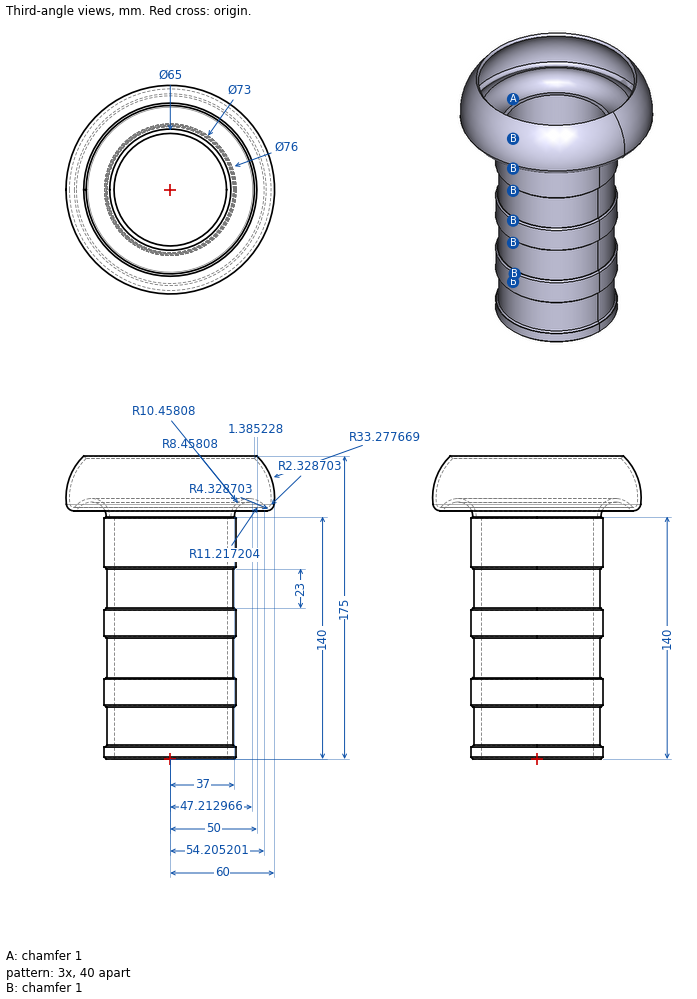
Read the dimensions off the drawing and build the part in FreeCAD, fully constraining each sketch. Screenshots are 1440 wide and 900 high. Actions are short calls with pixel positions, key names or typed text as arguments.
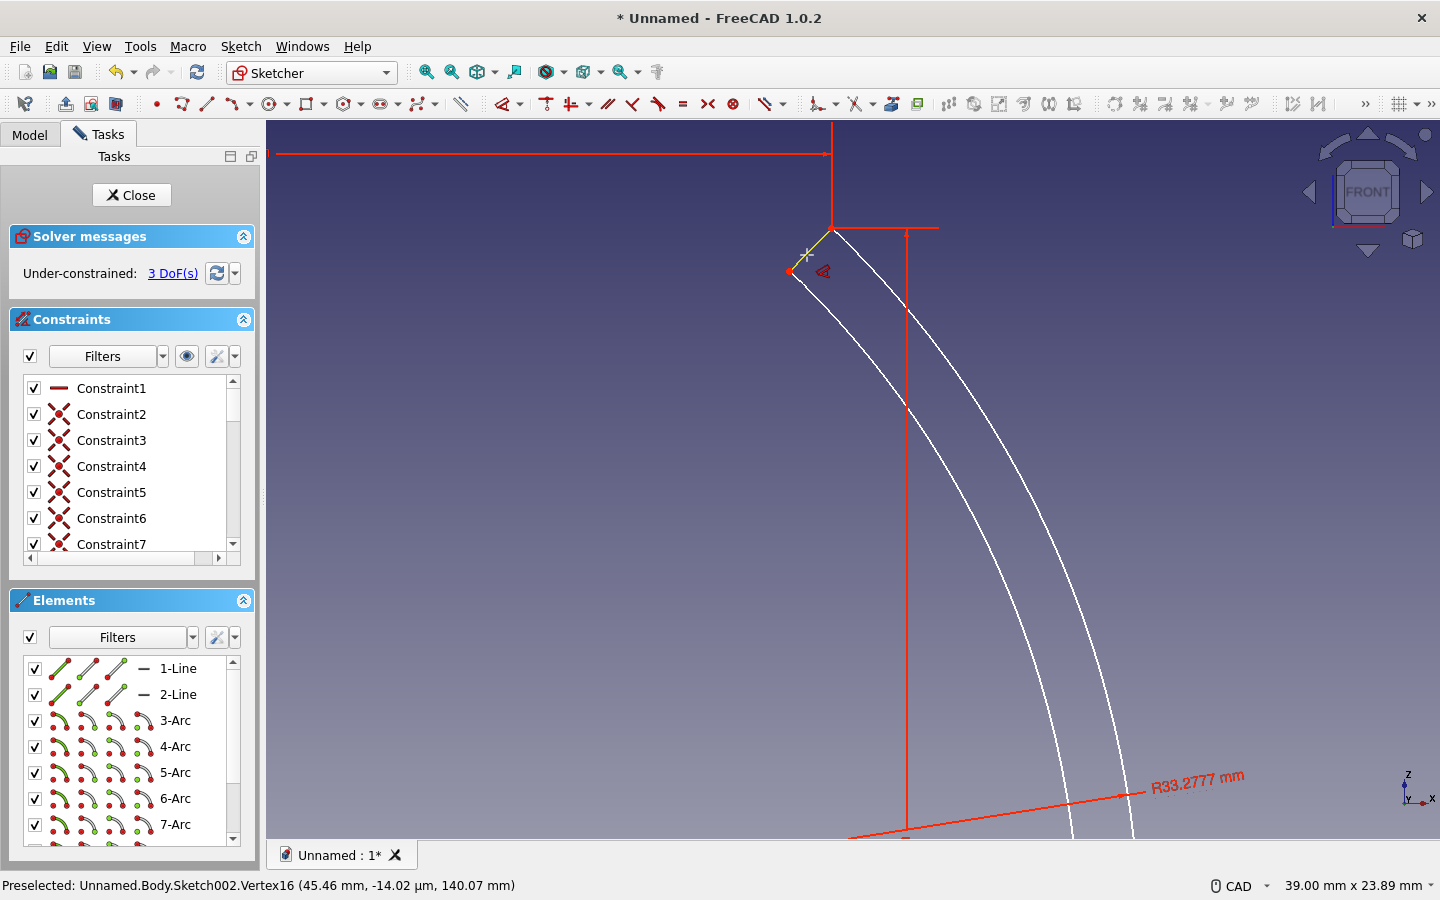
click(807, 254)
click(811, 194)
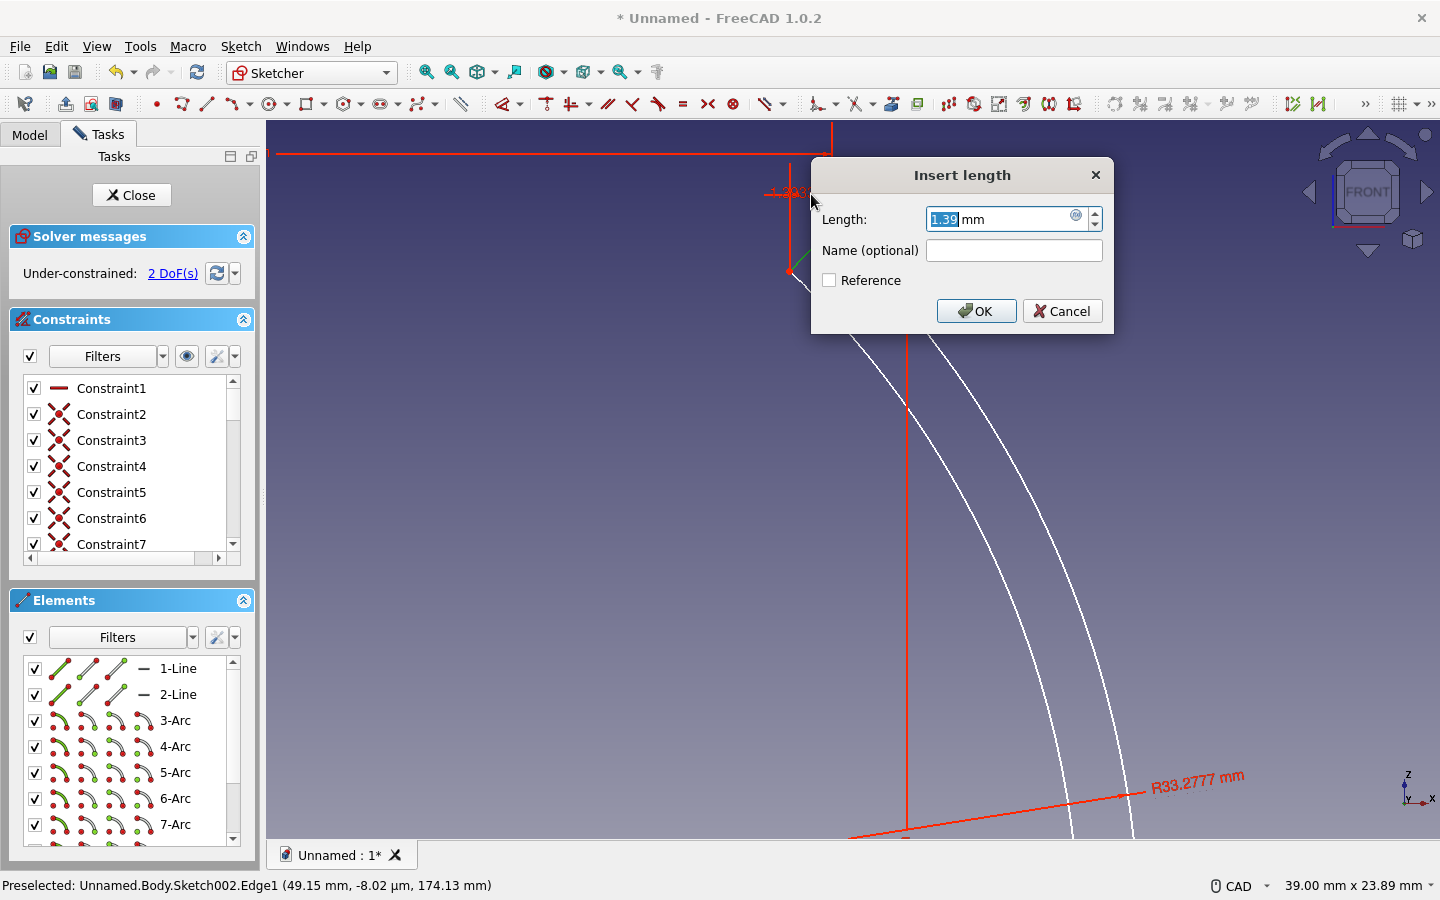
text(1.385228)
key(Return)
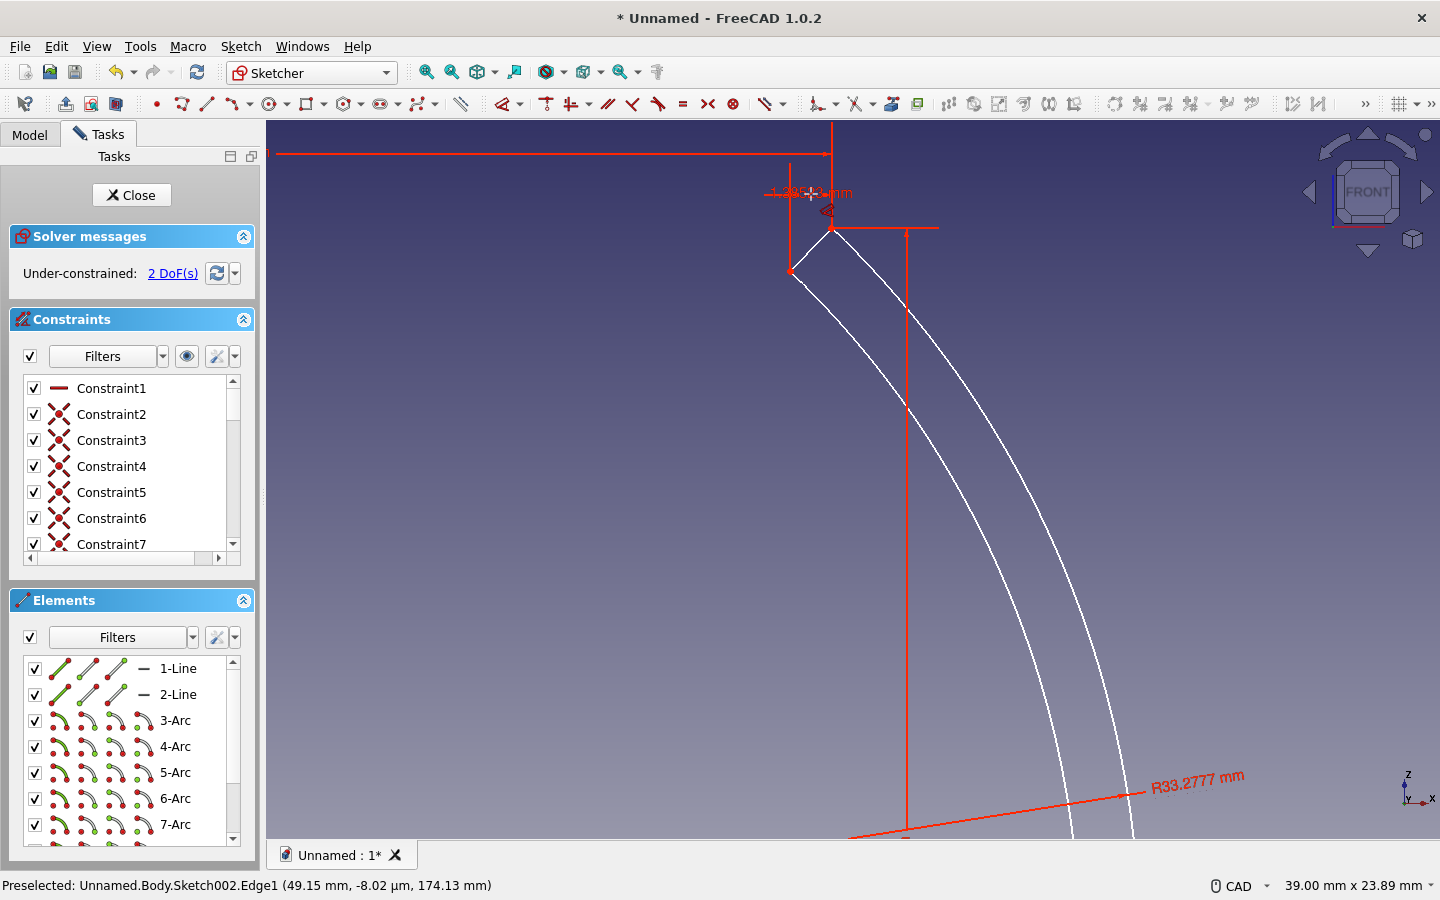
scroll(807, 255, down, 4)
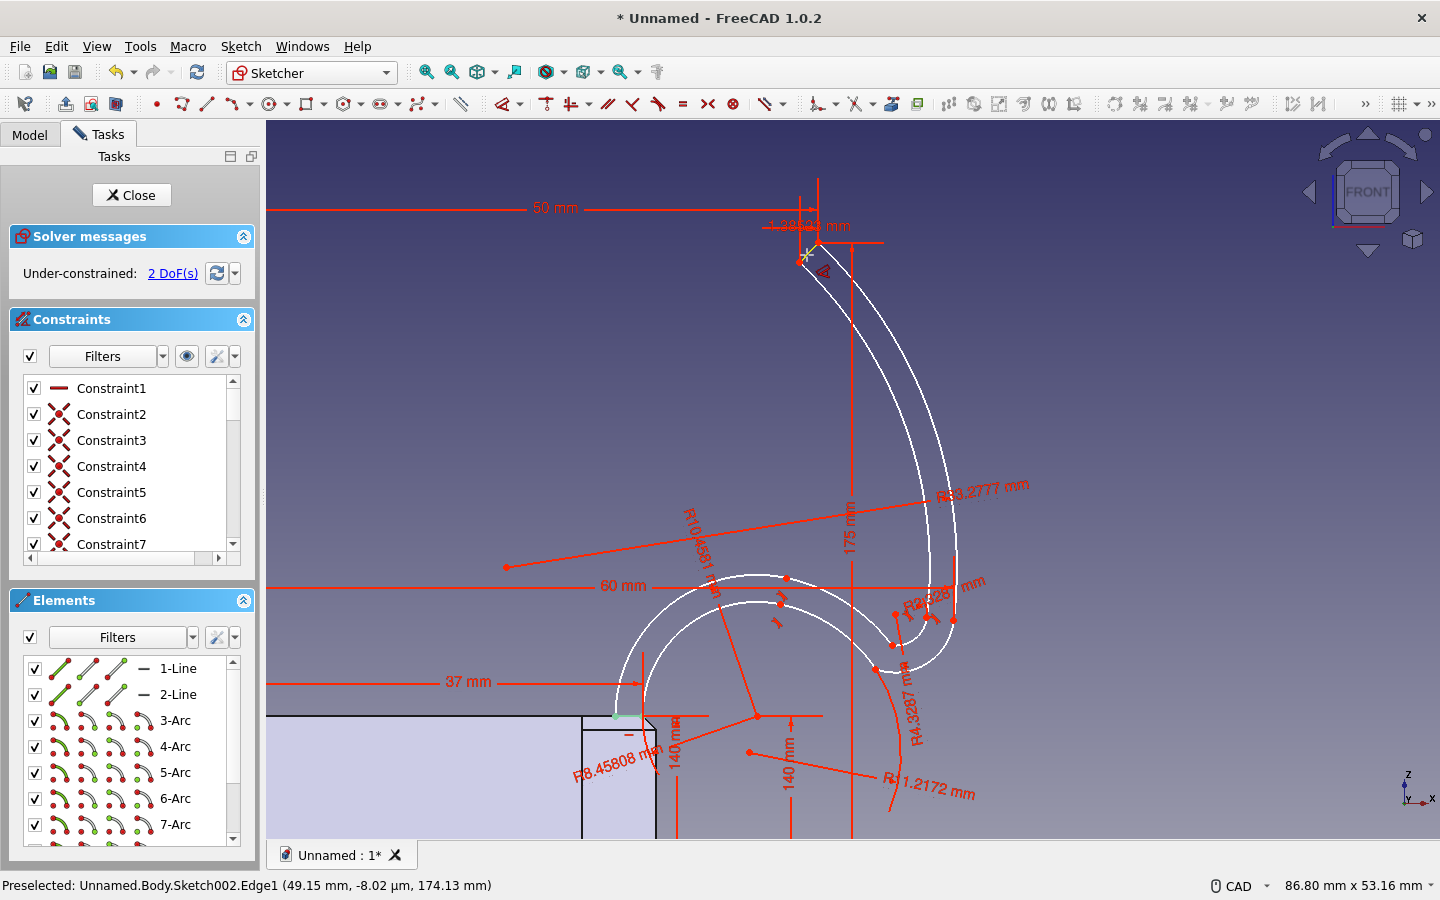
click(876, 669)
click(585, 635)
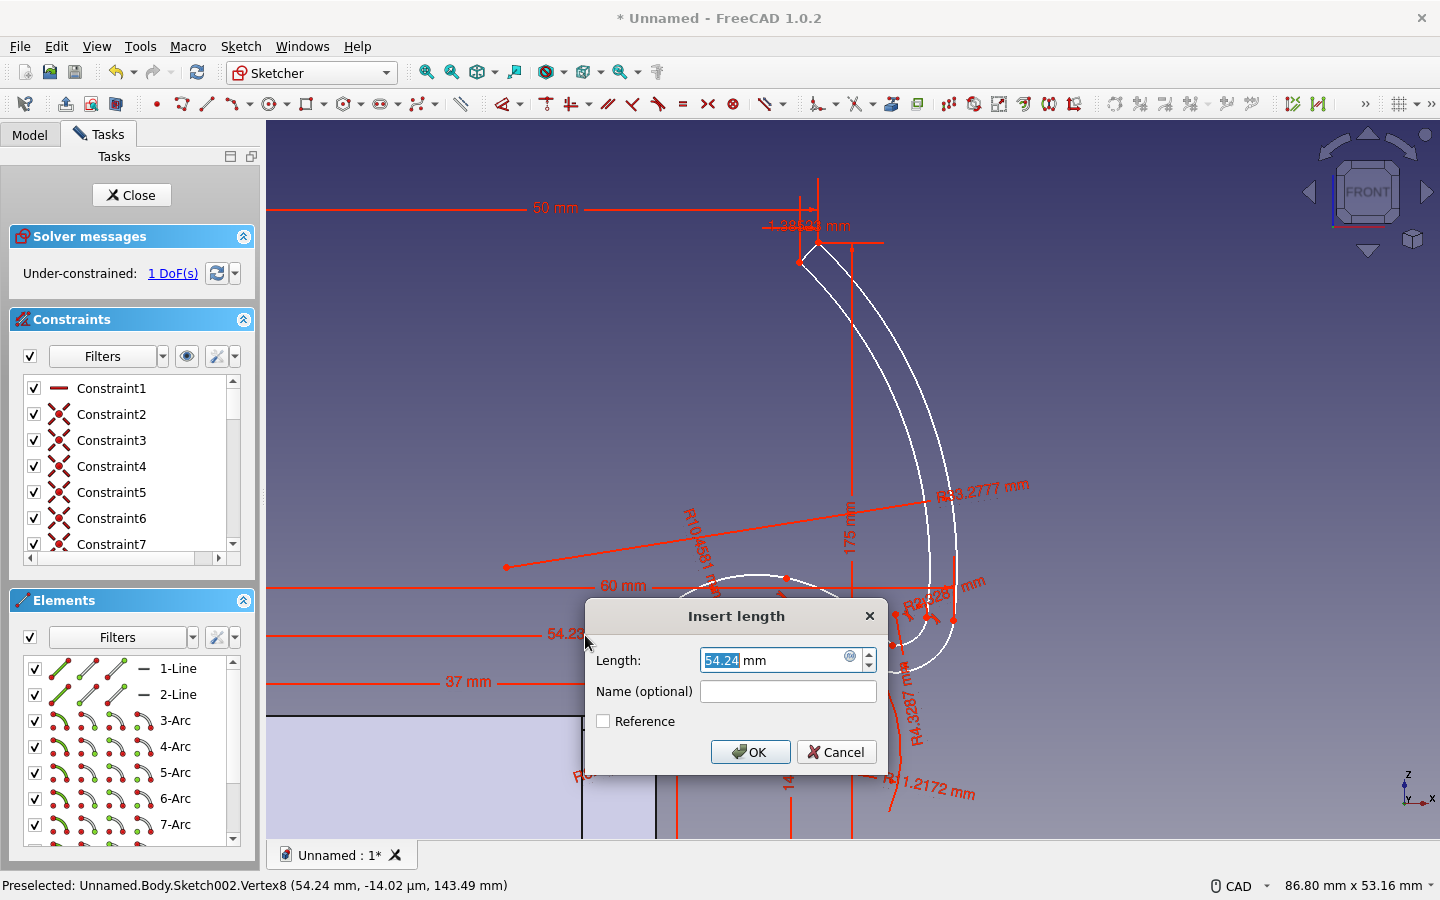
text(54.205201)
key(Return)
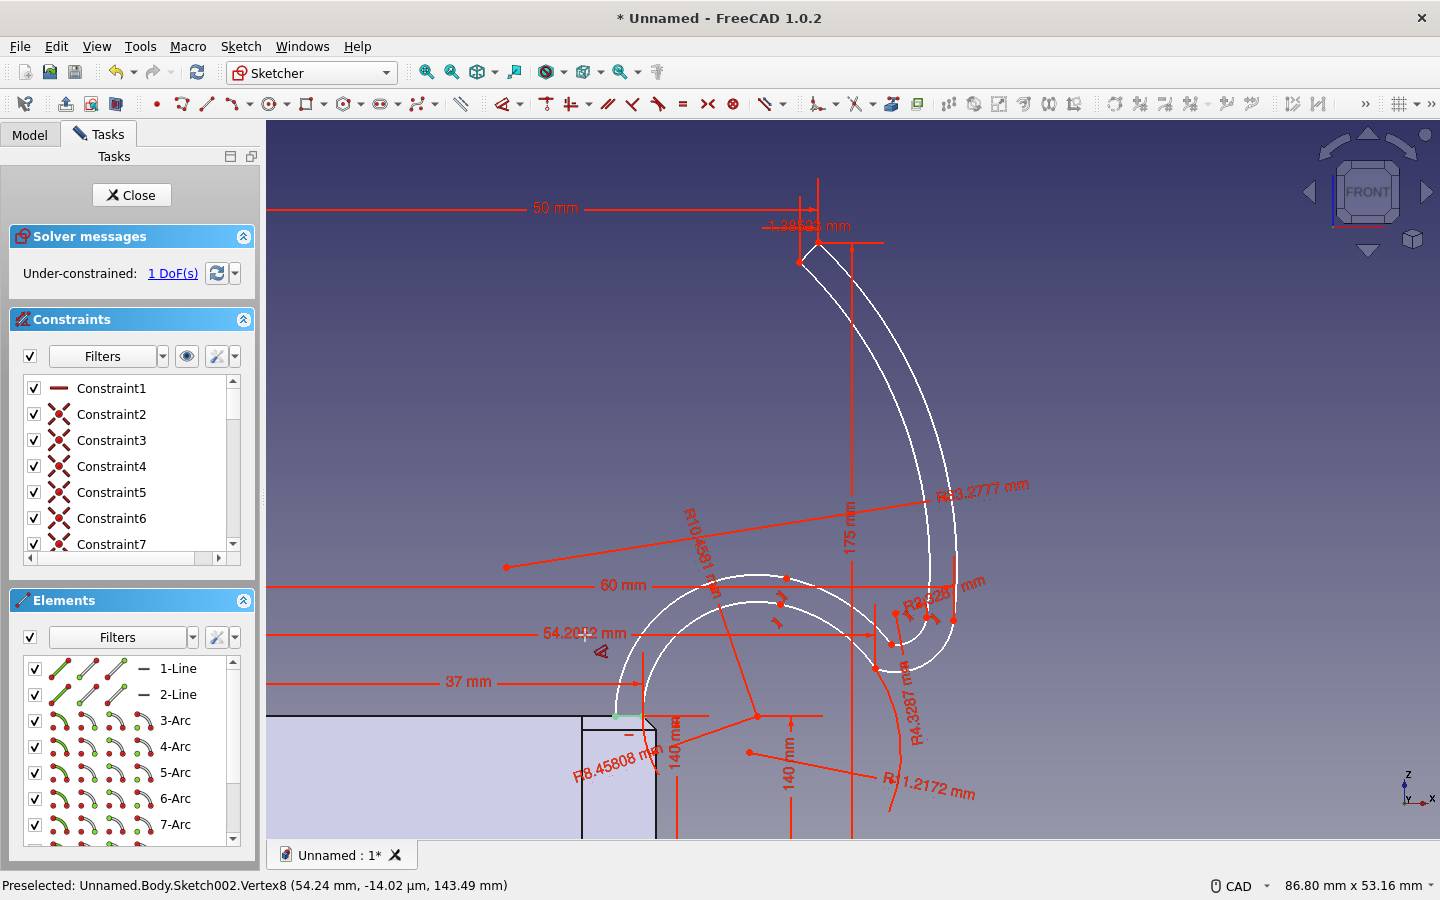
click(781, 604)
click(537, 570)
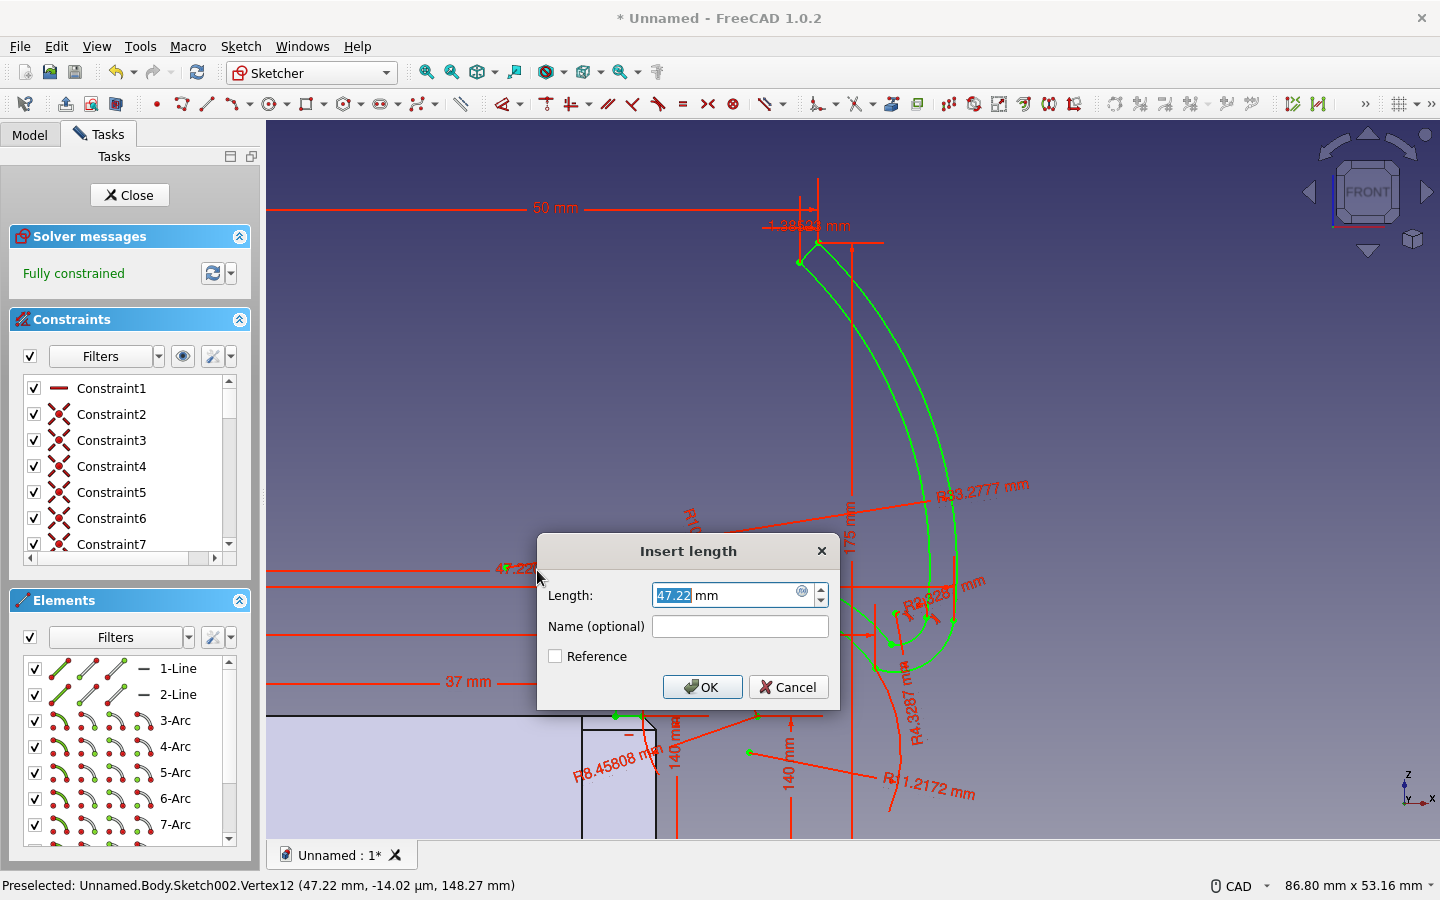
text(47.212966)
key(Return)
key(Escape)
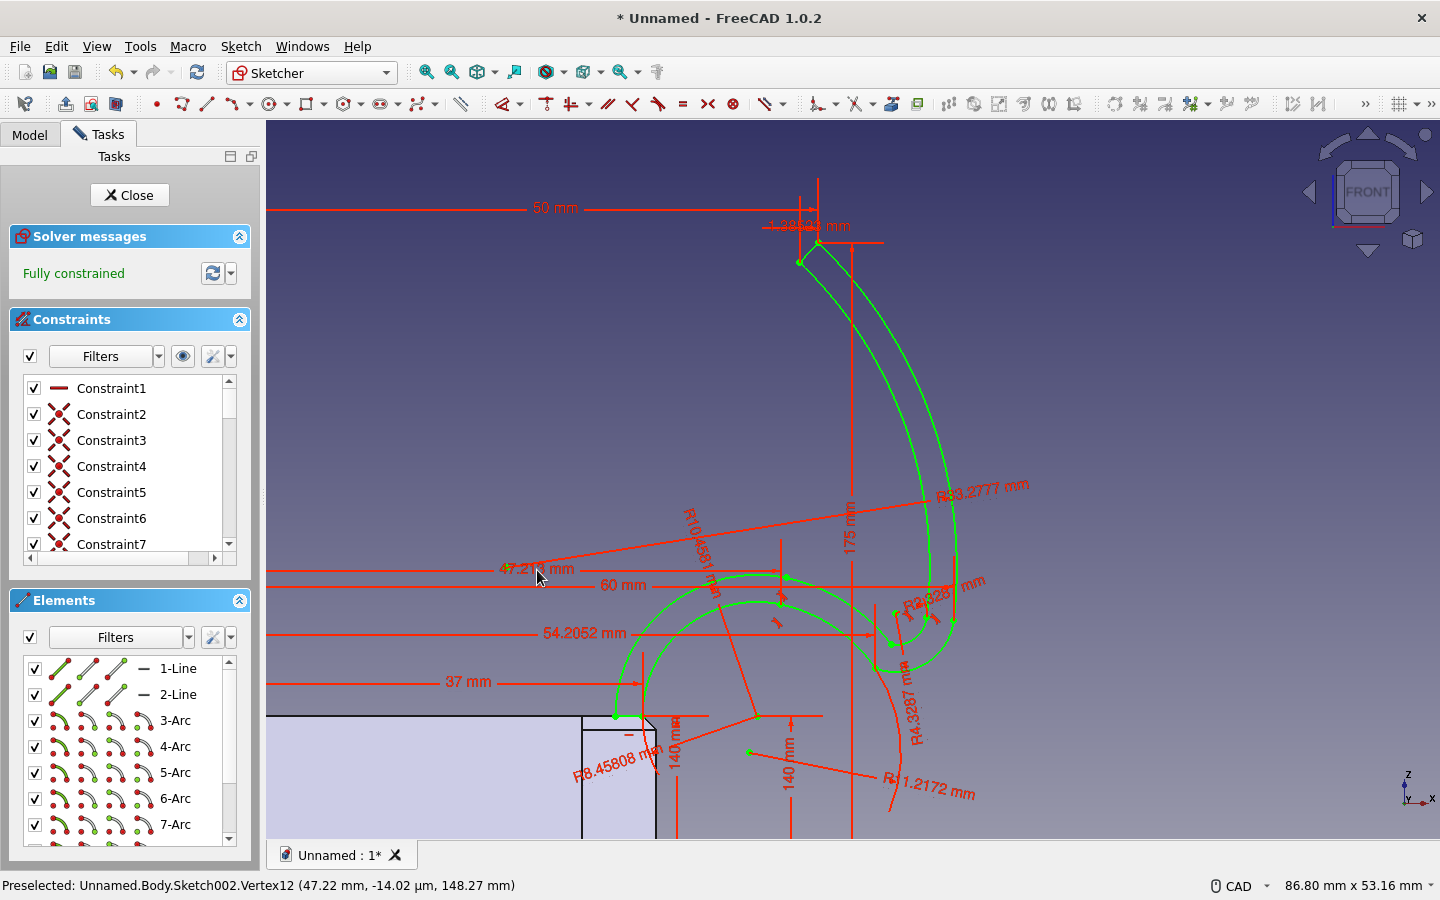
click(130, 195)